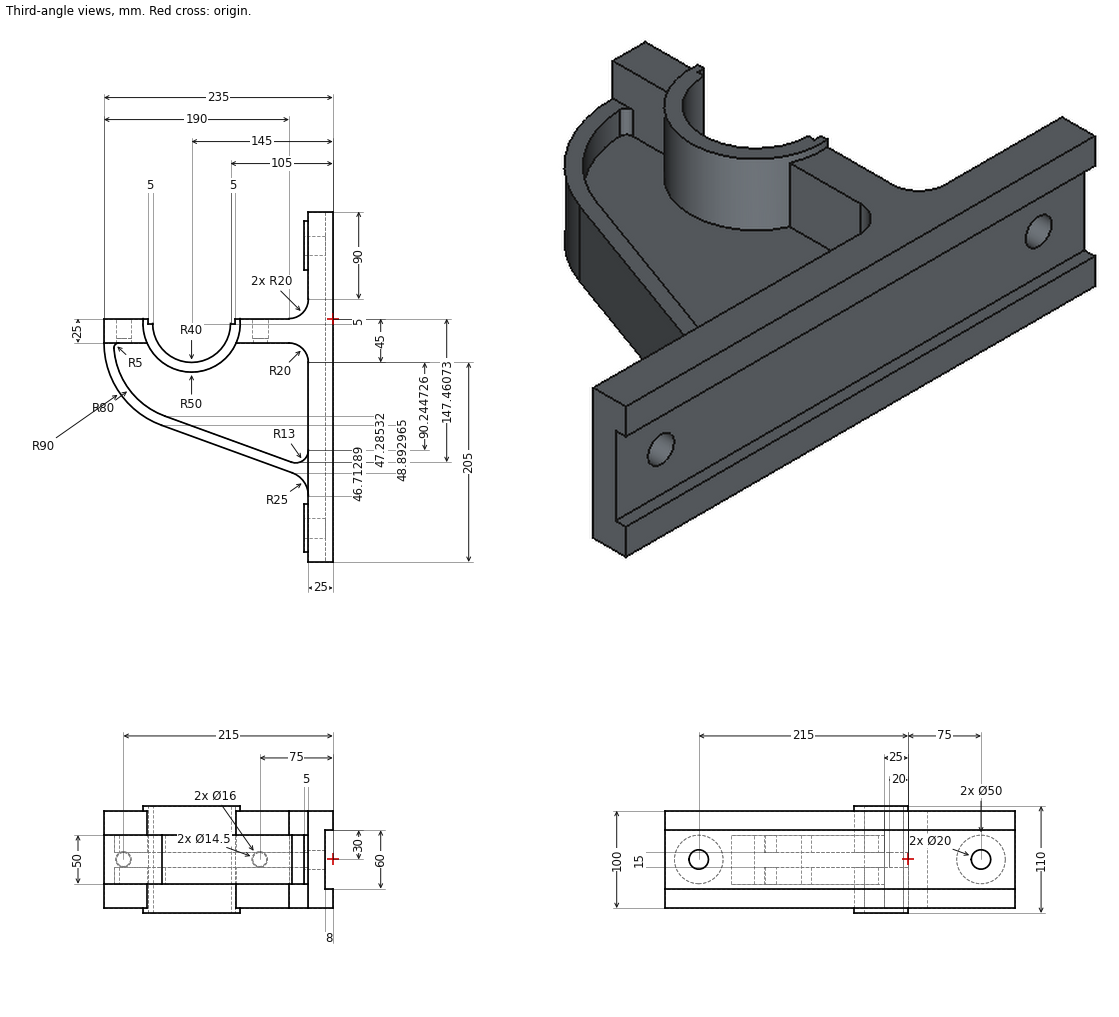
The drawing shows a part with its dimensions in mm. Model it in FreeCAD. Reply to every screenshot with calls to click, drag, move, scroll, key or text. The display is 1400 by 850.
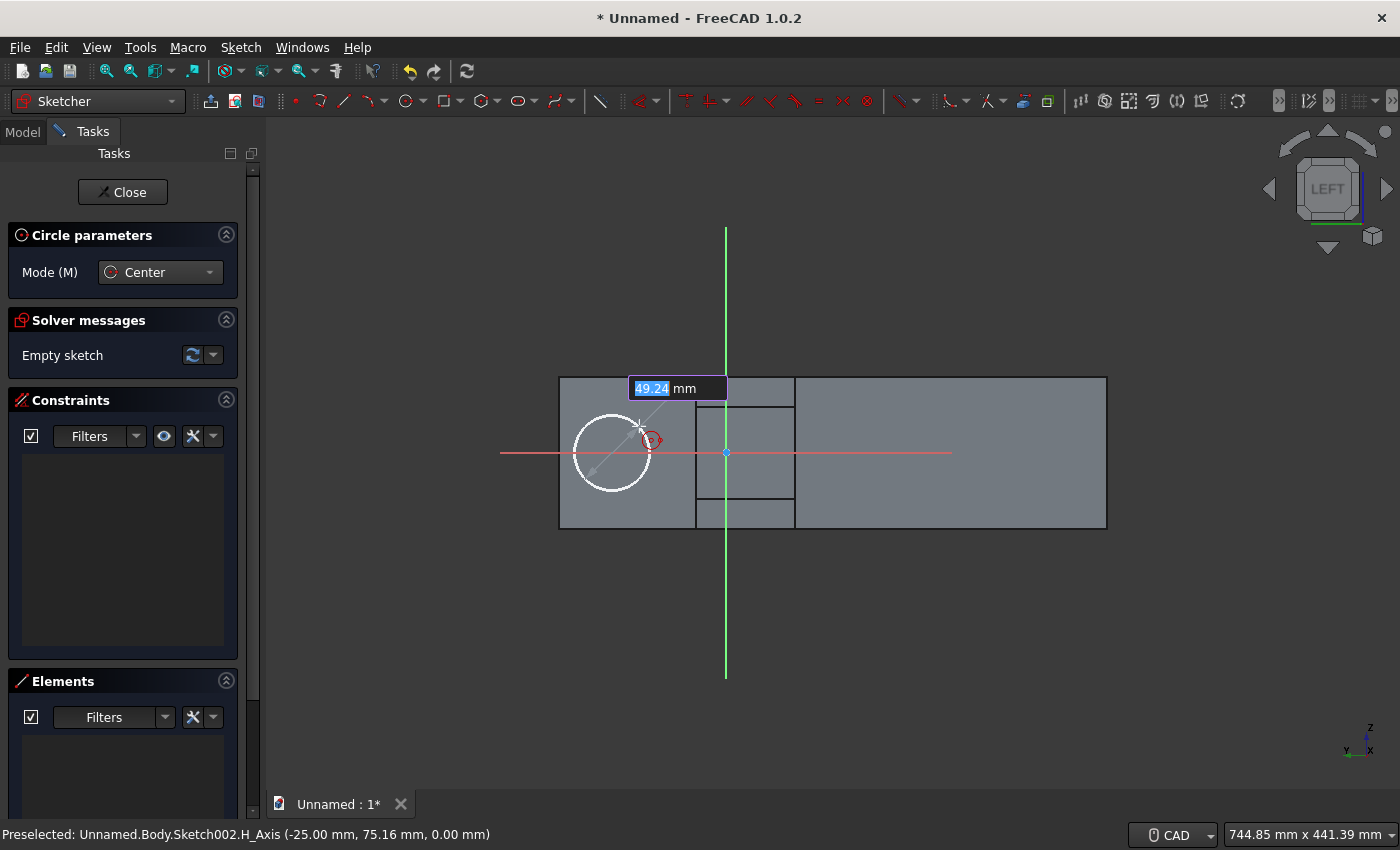
text(50)
key(Return)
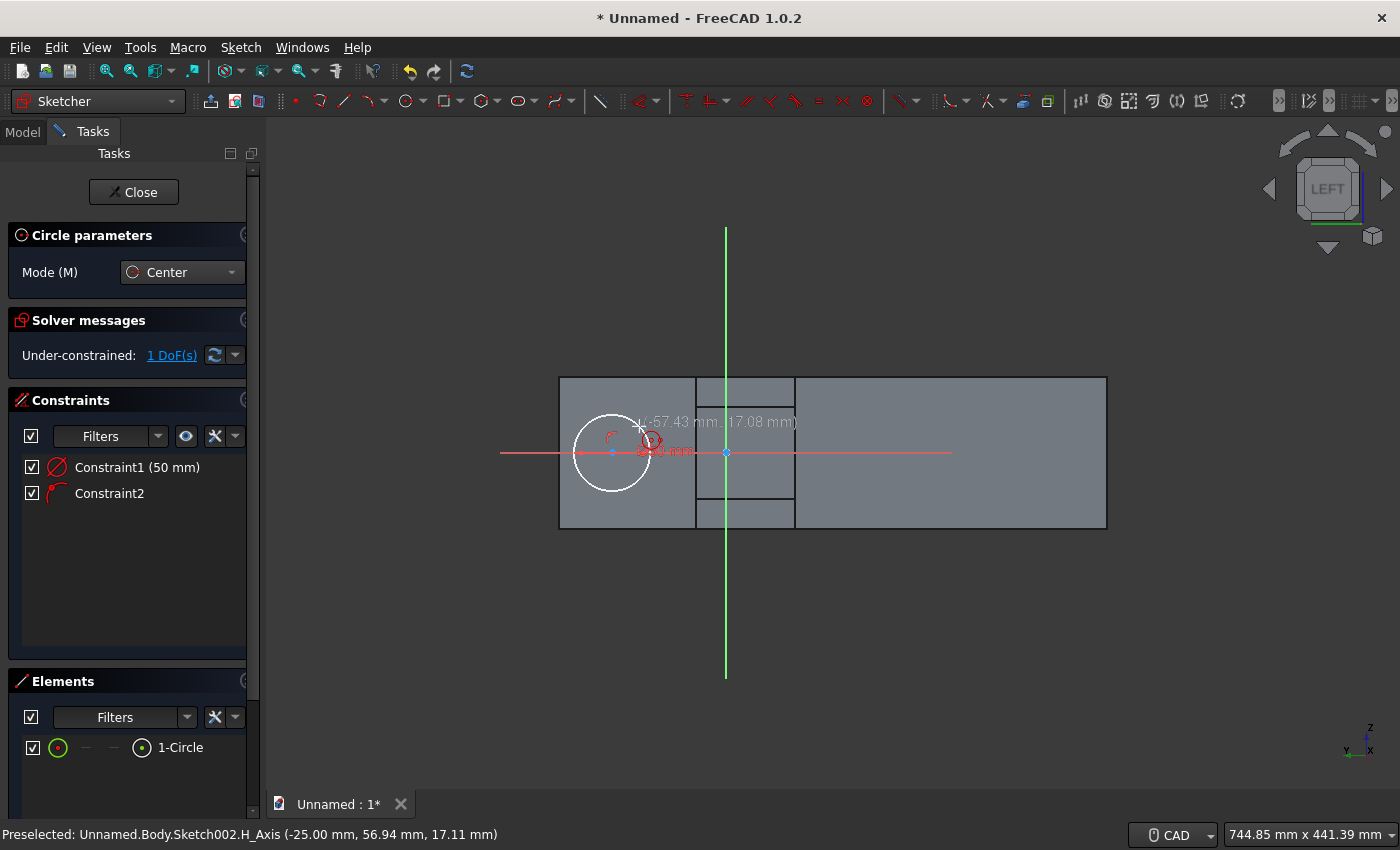
click(1054, 453)
move(1081, 426)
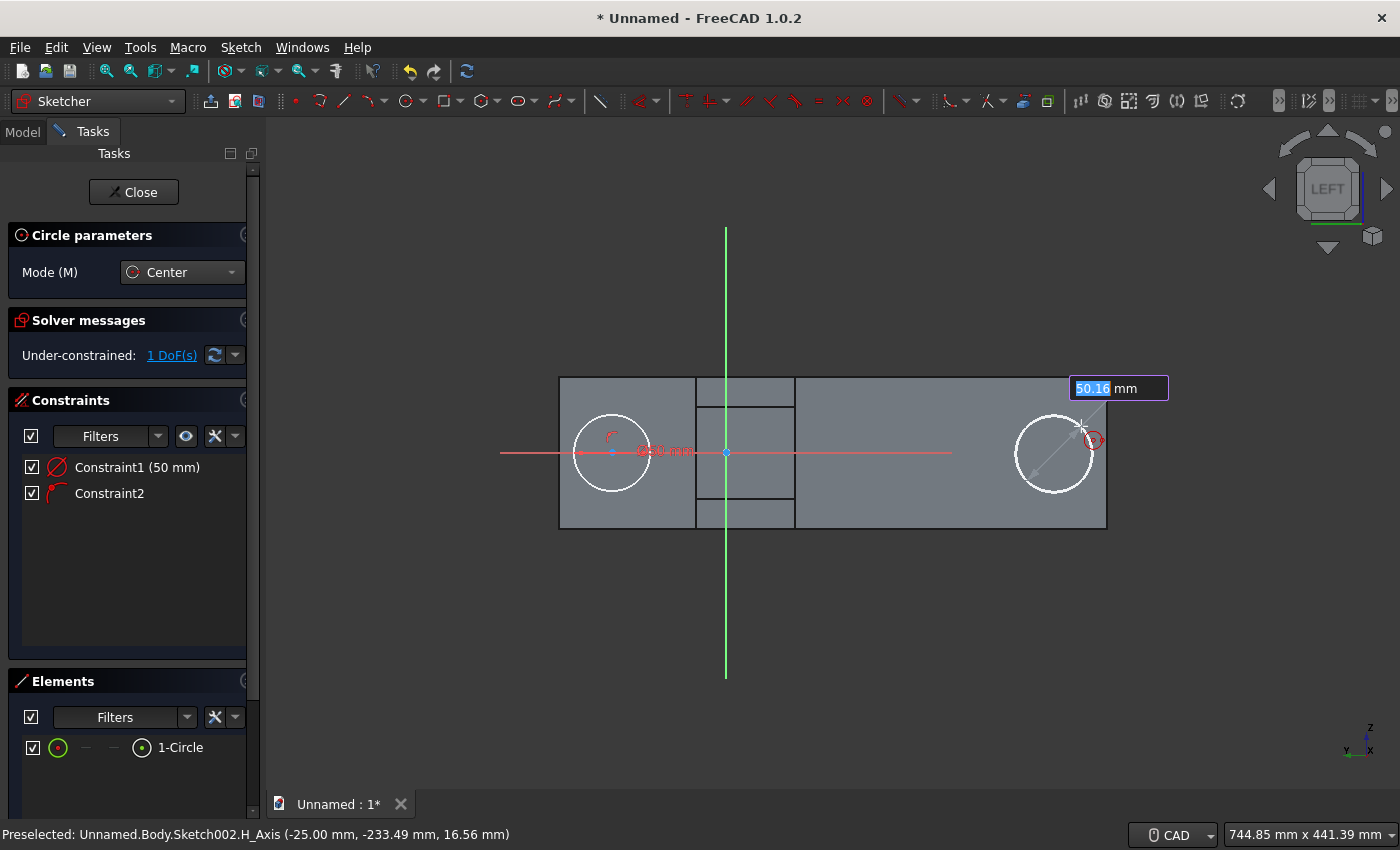
text(50)
key(Return)
key(Escape)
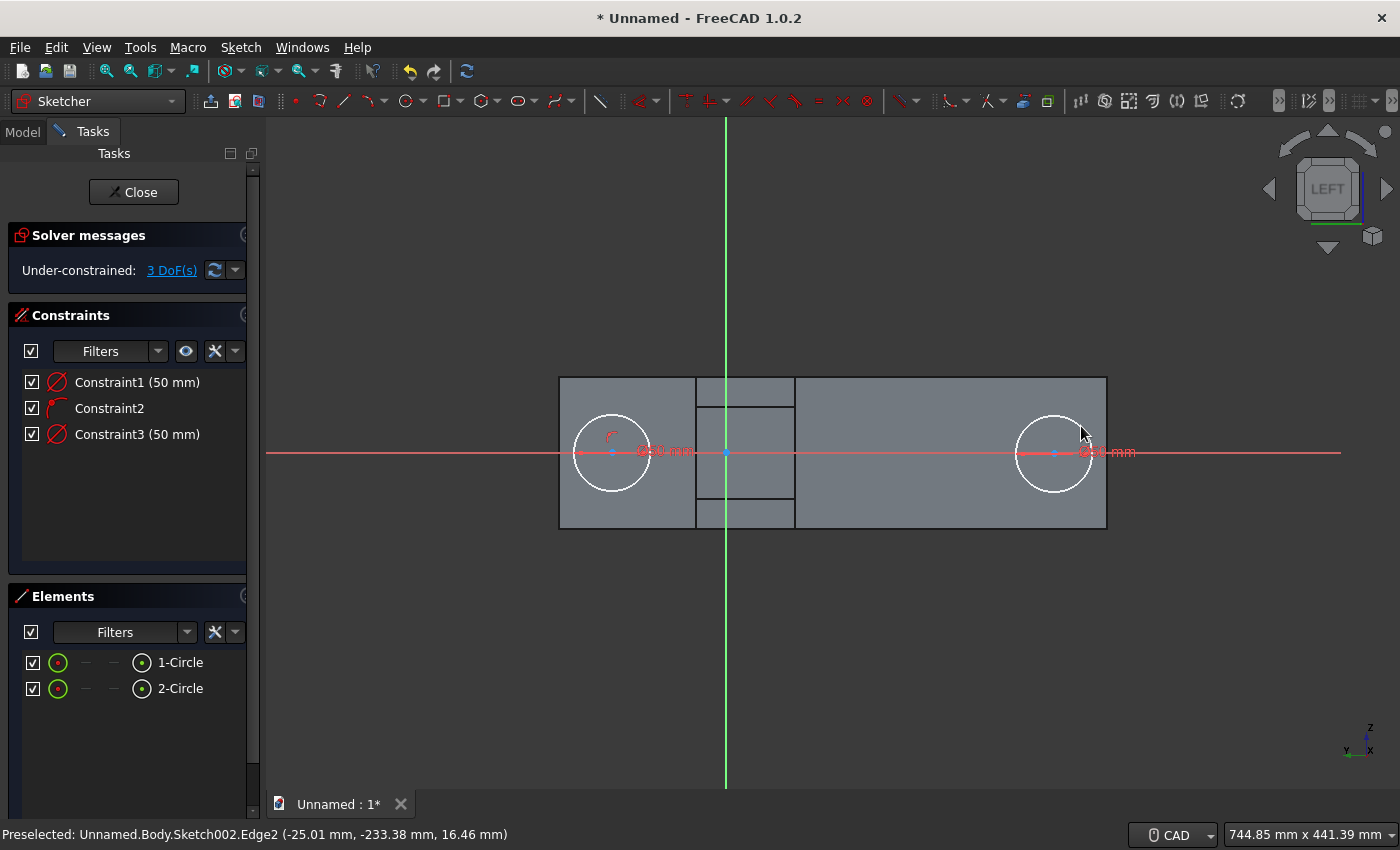
click(1054, 454)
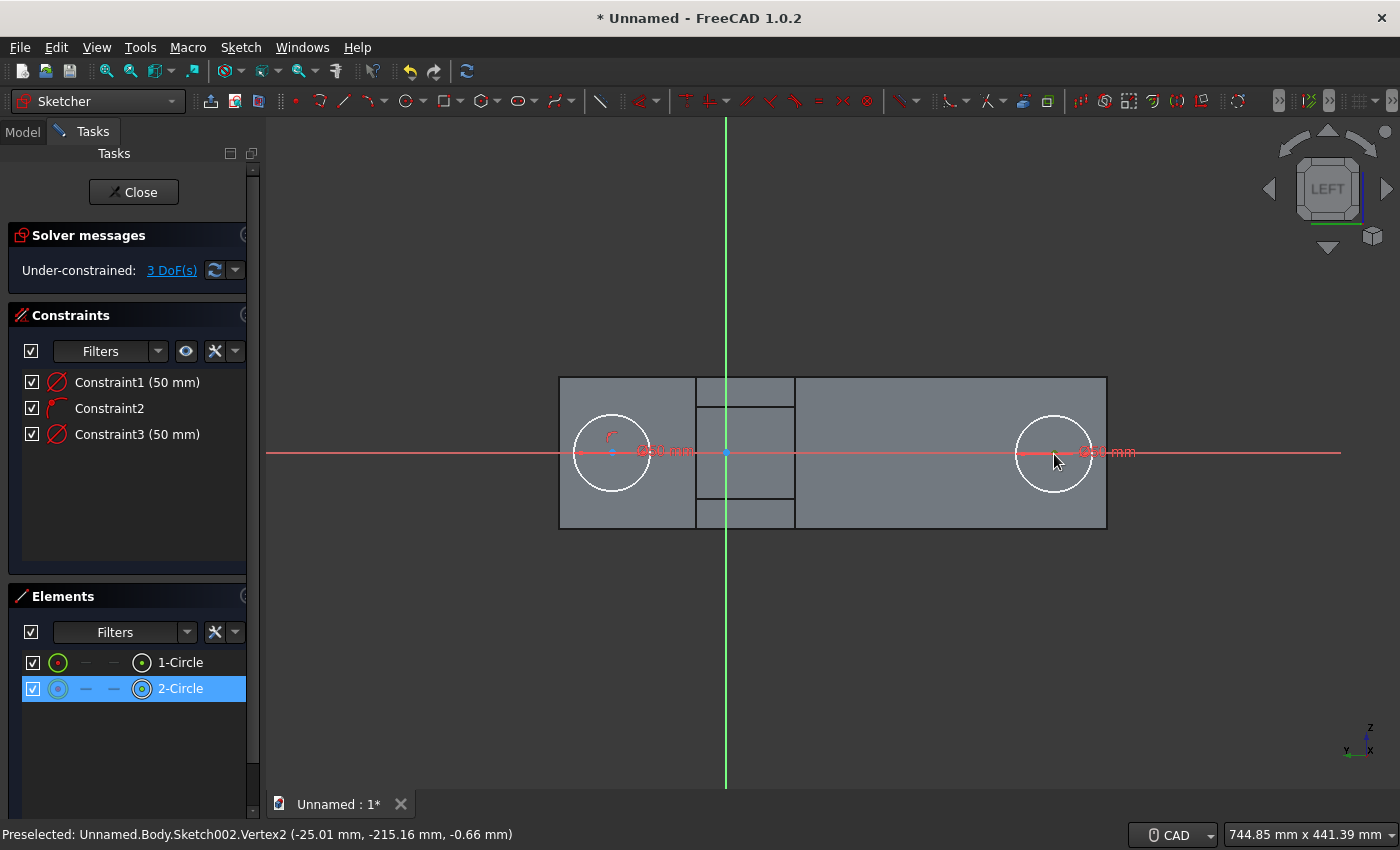
click(361, 453)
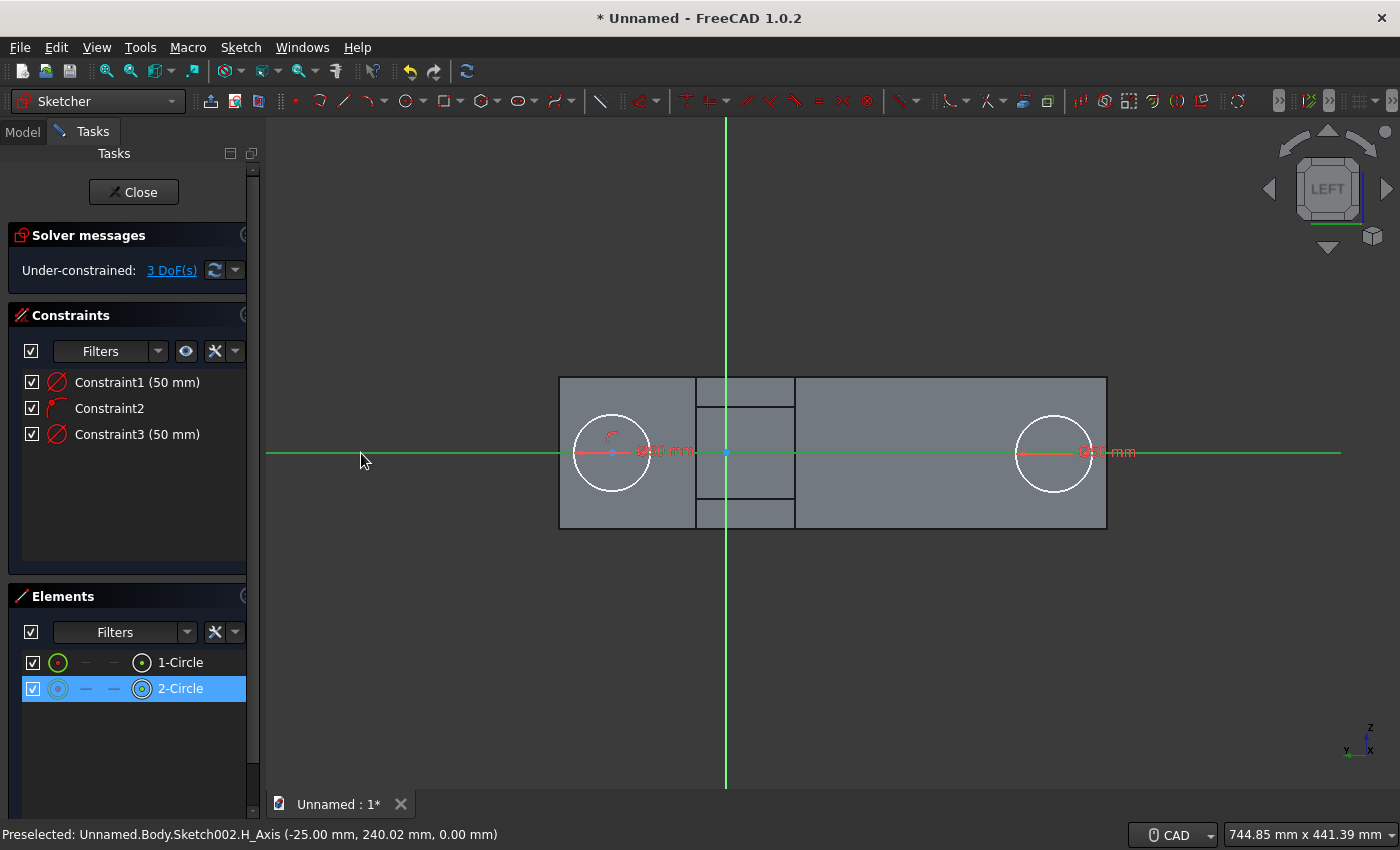
click(686, 102)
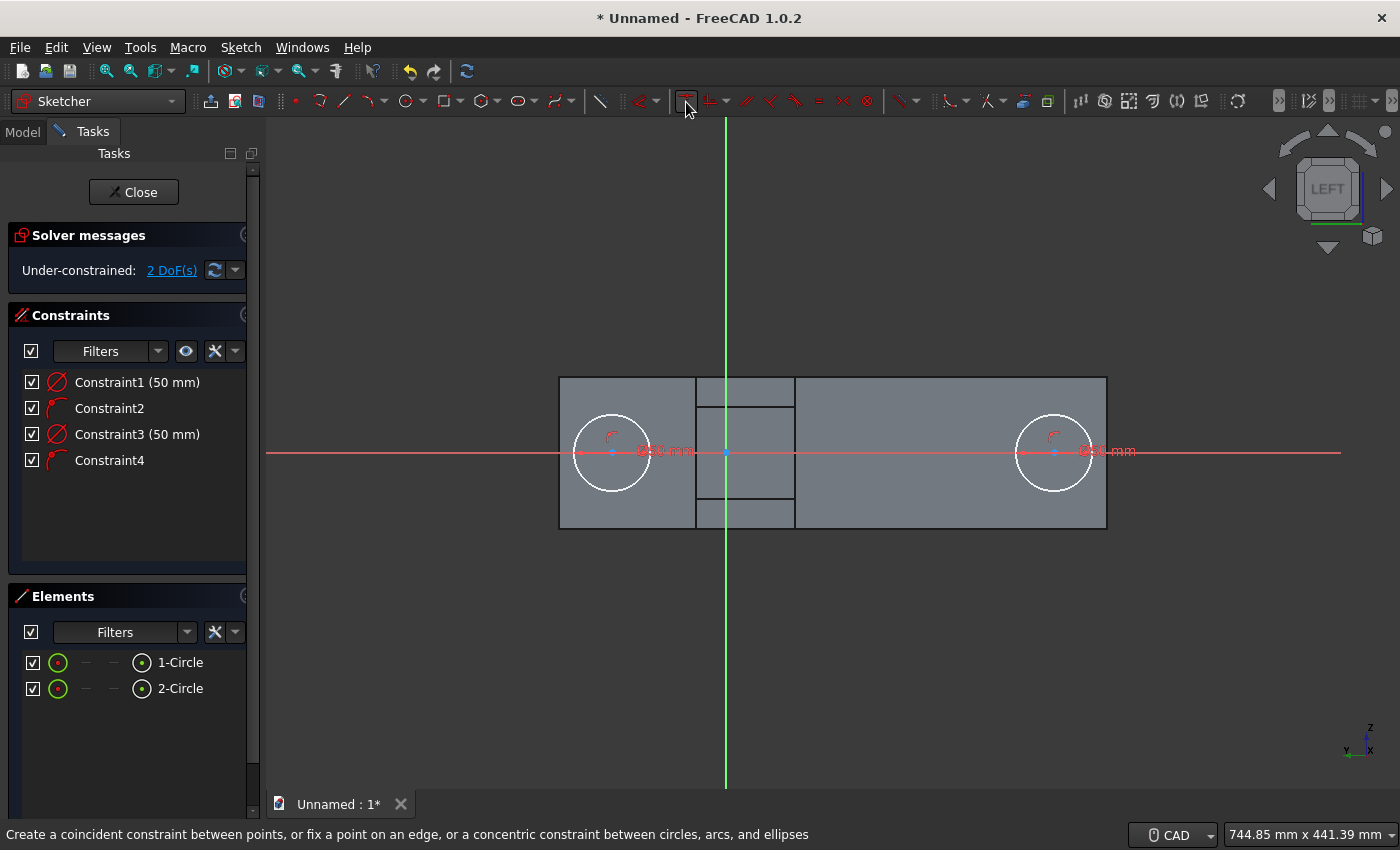
click(640, 102)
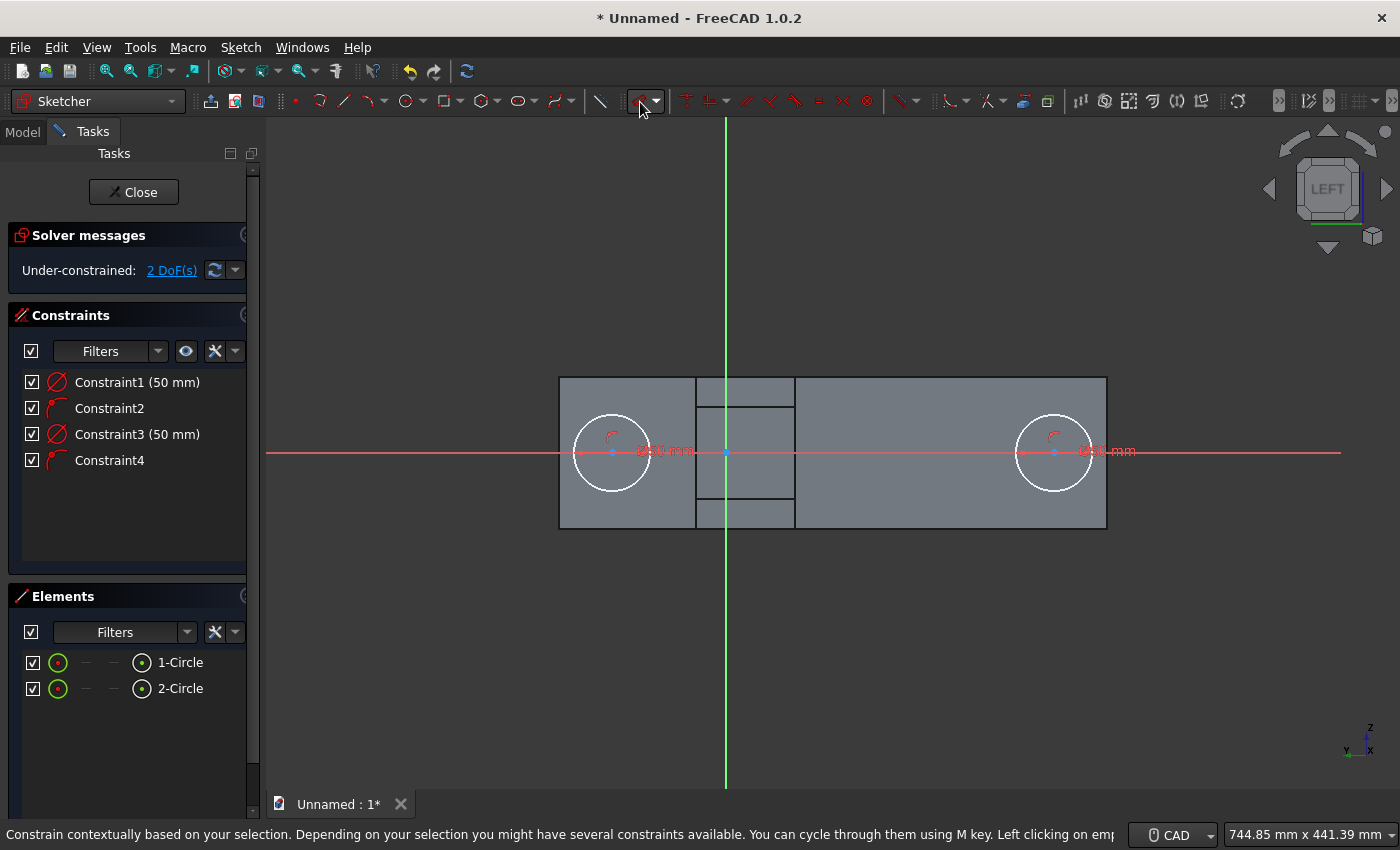
click(612, 453)
click(669, 487)